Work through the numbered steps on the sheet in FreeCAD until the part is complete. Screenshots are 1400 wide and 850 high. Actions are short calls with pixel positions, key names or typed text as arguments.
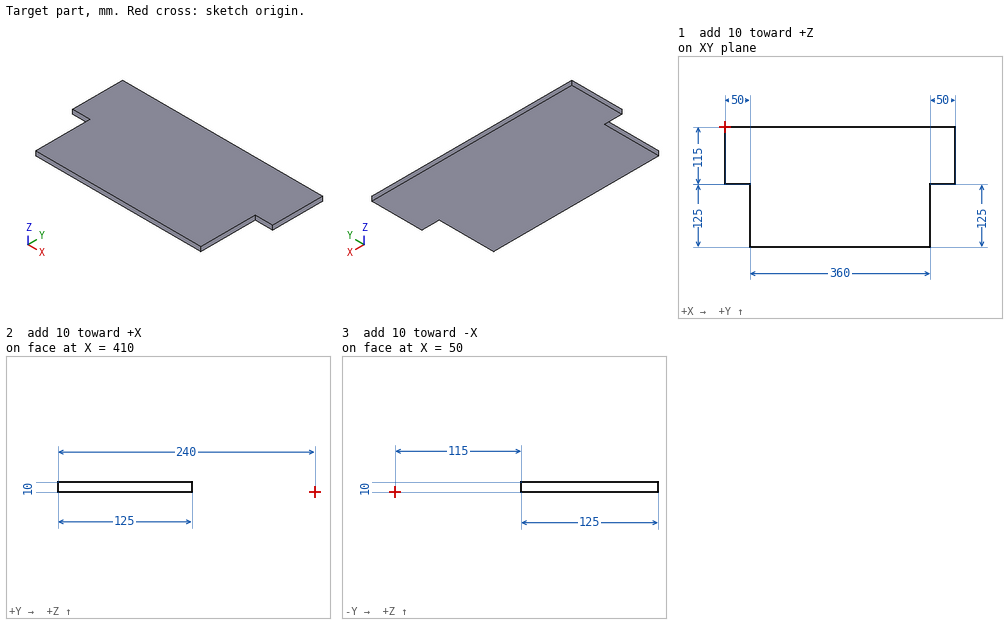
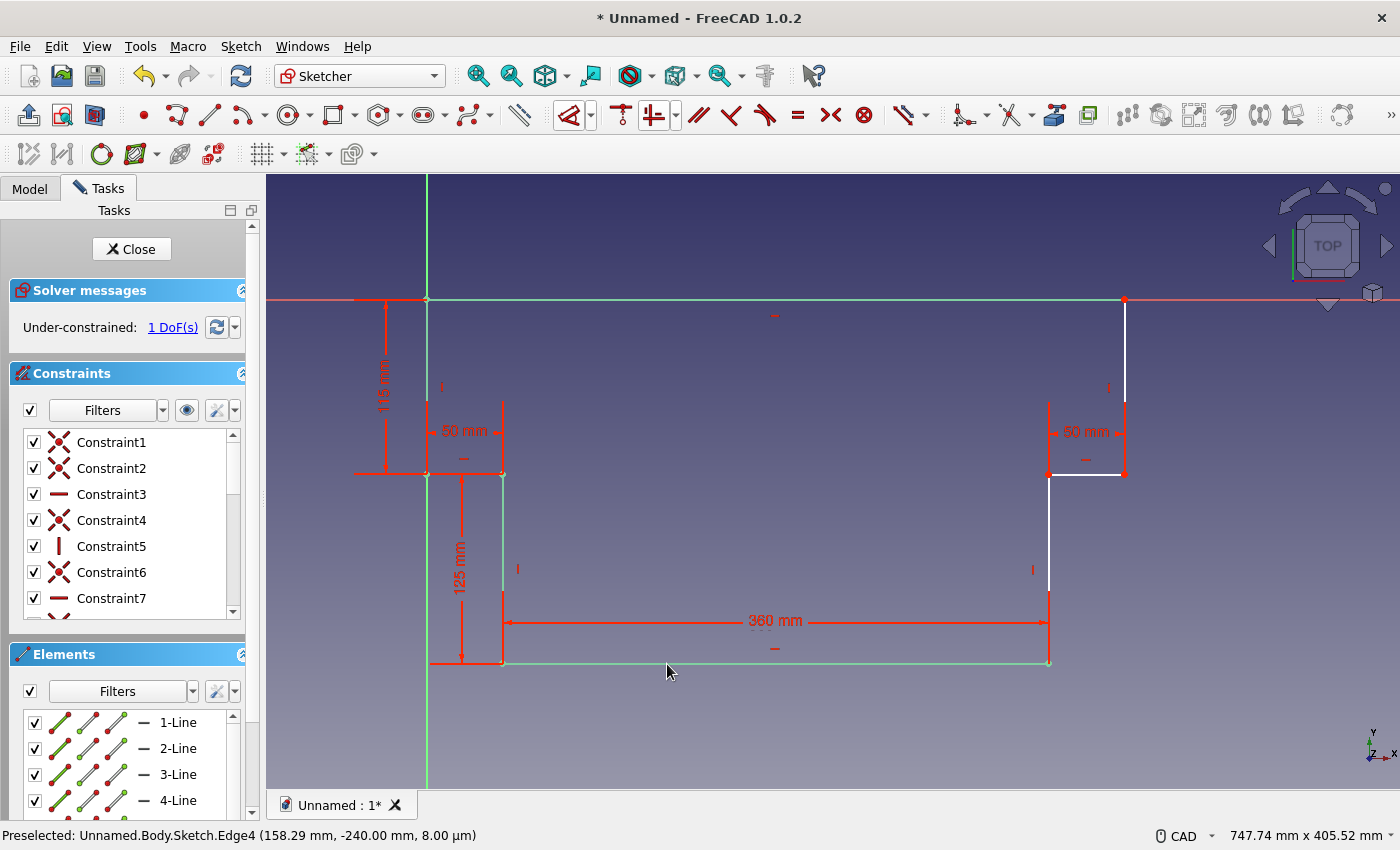
click(1049, 607)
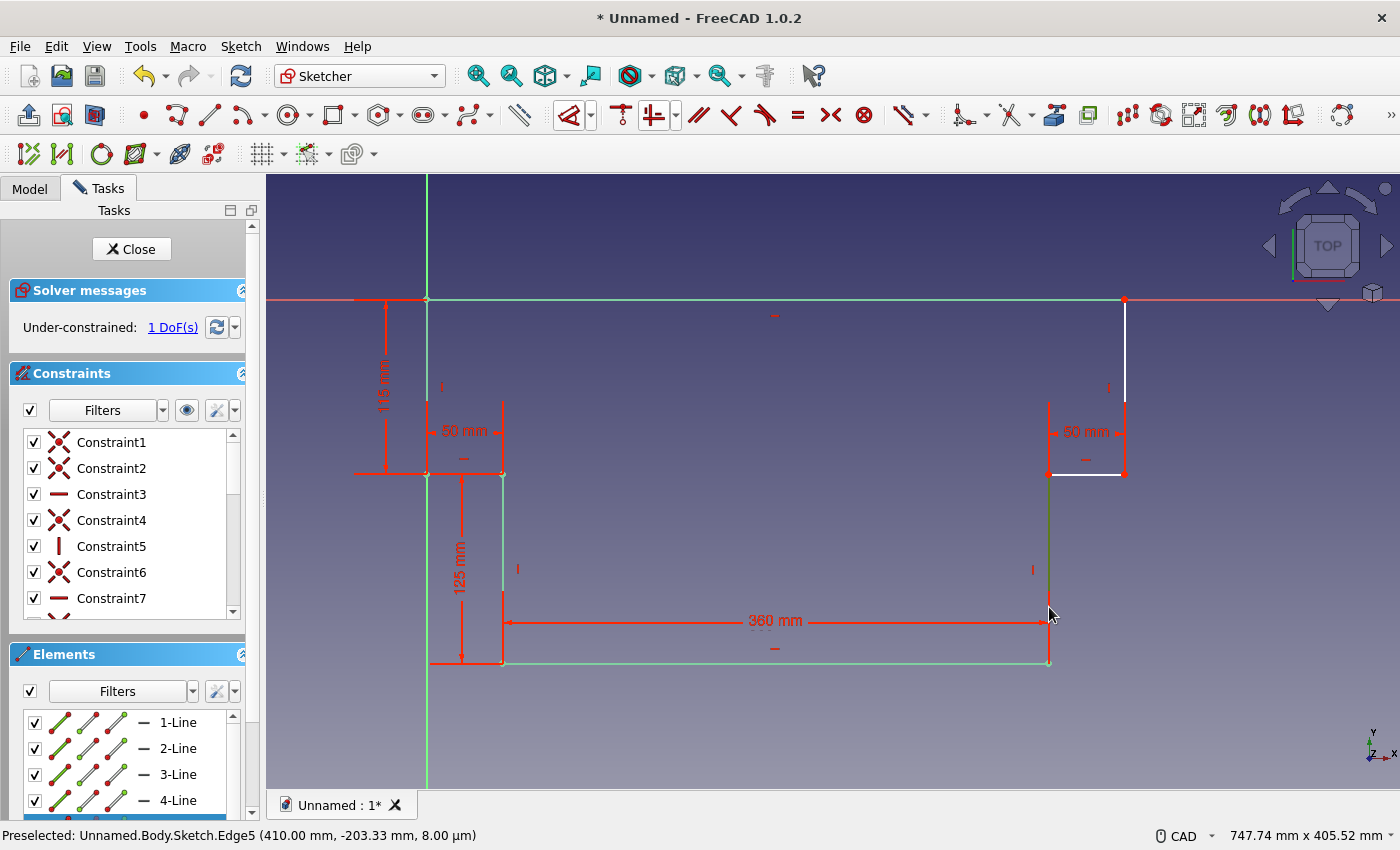
key(i)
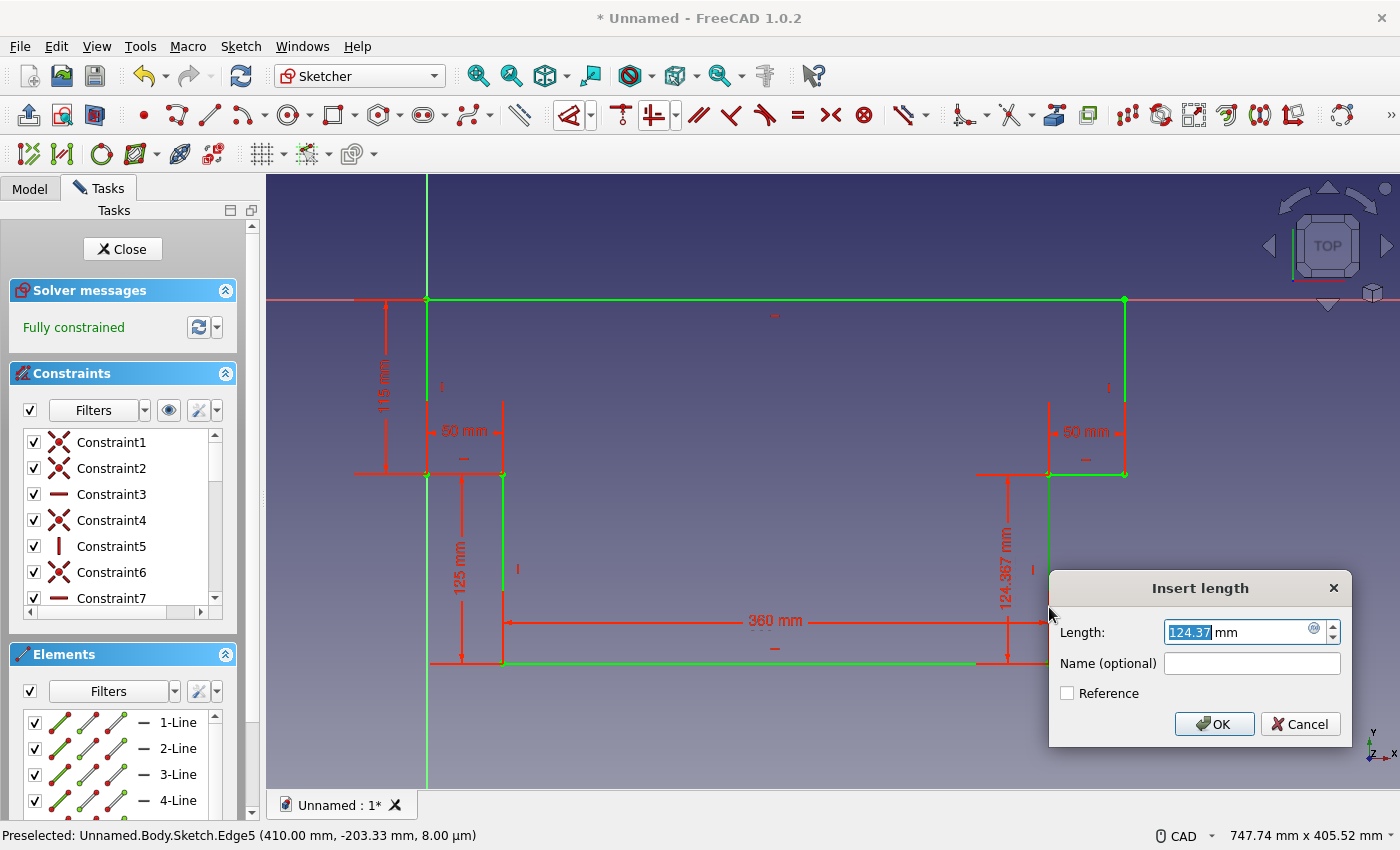
text(125)
key(Return)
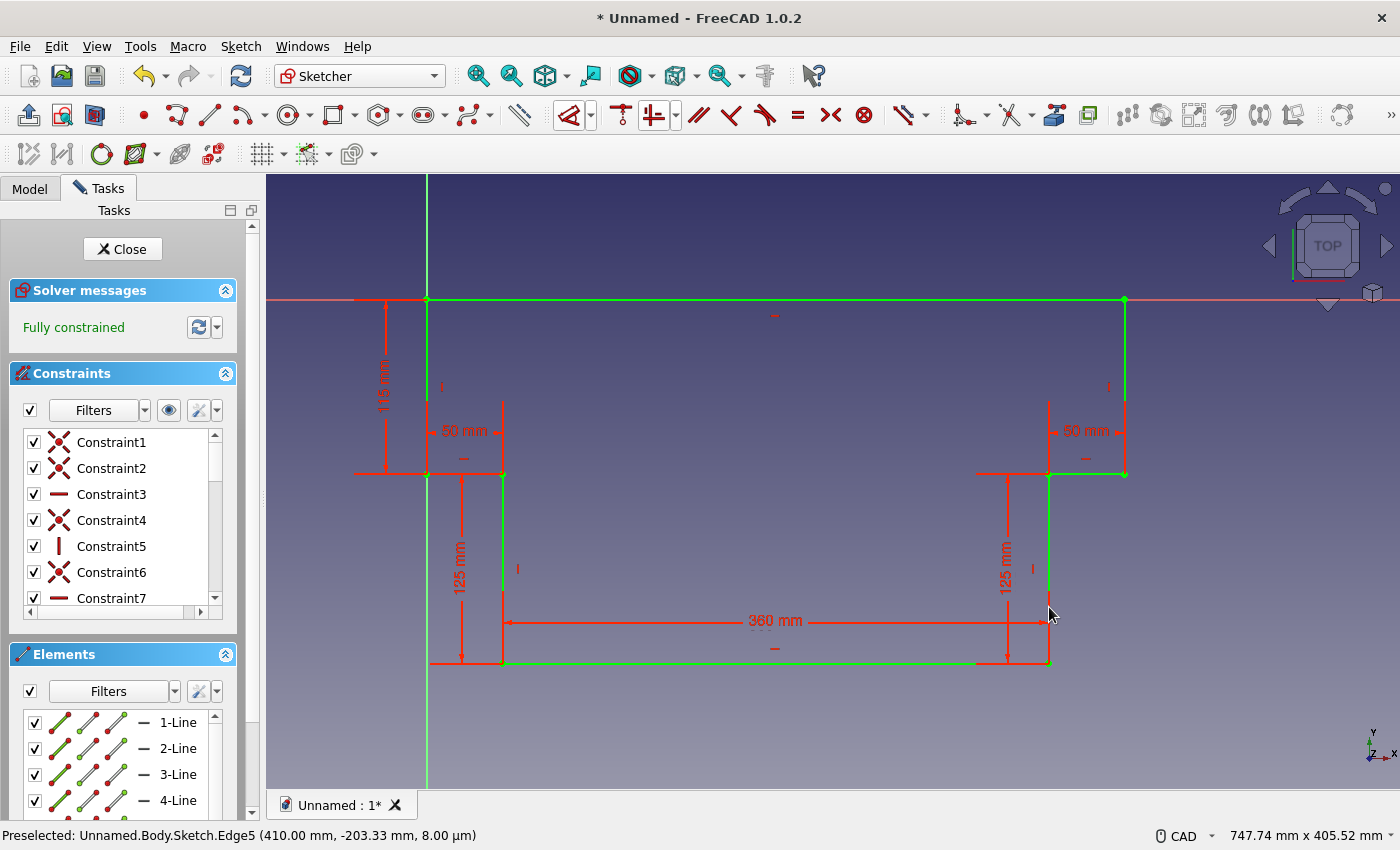
click(123, 249)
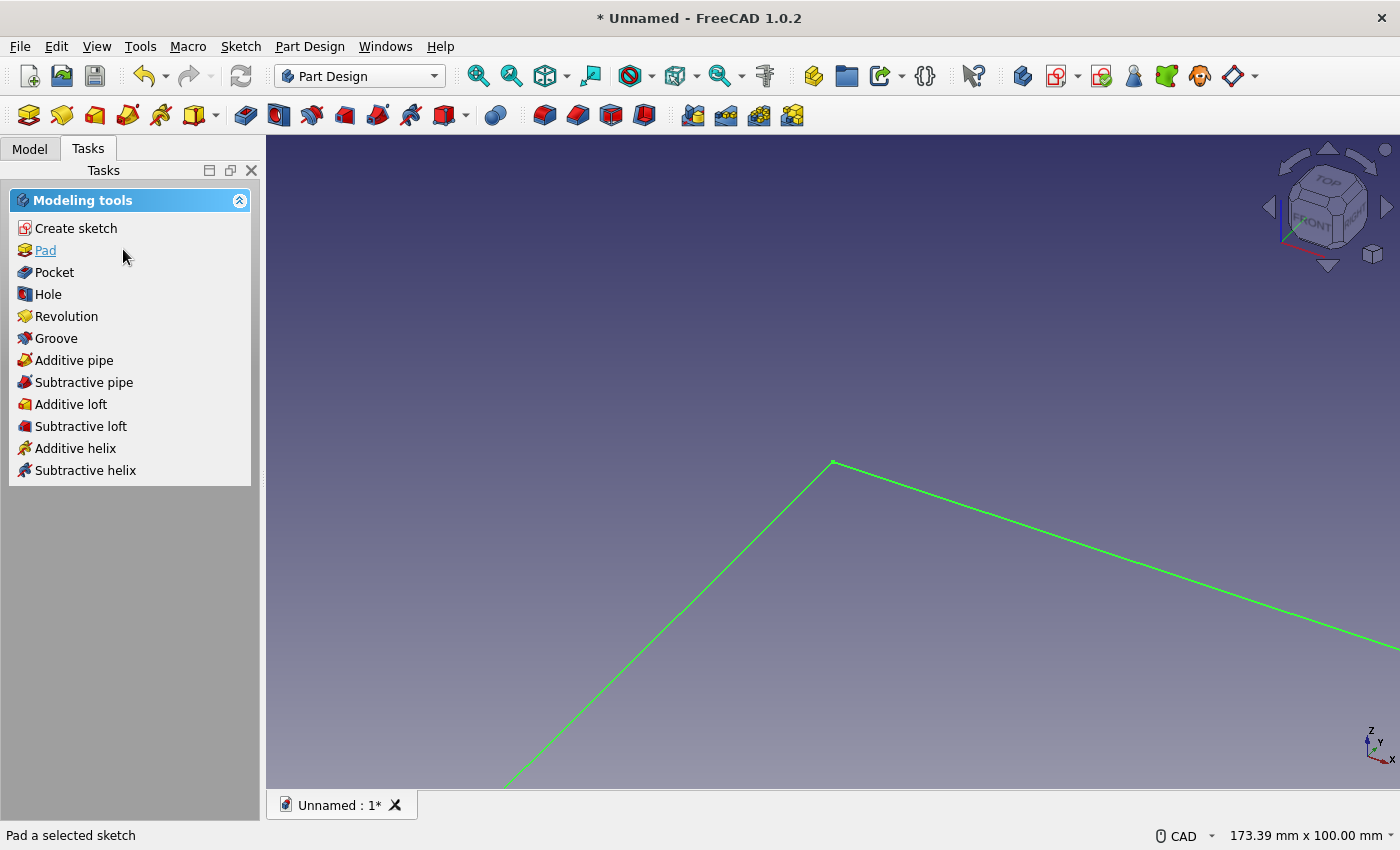
click(29, 116)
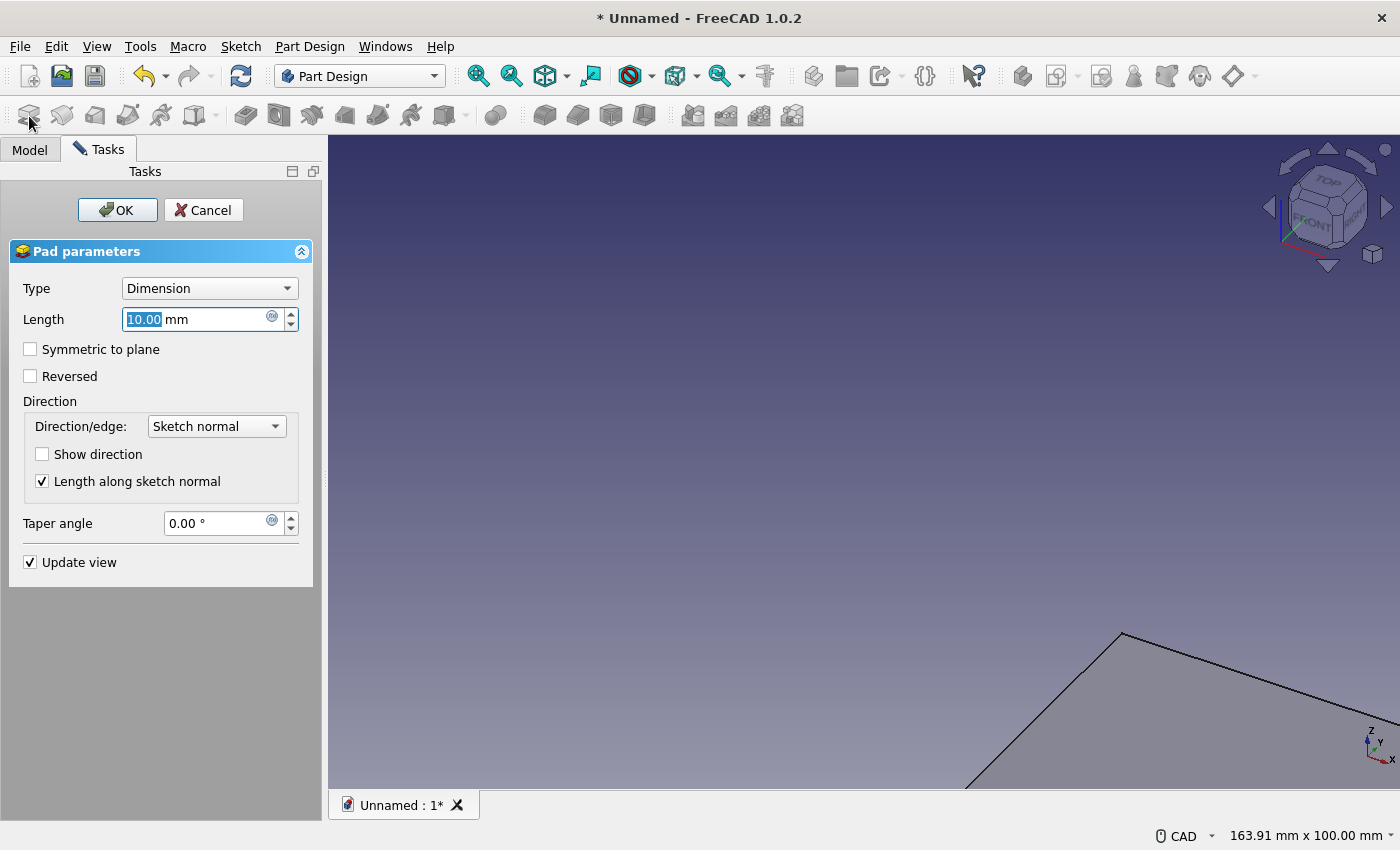
text(10)
key(Tab)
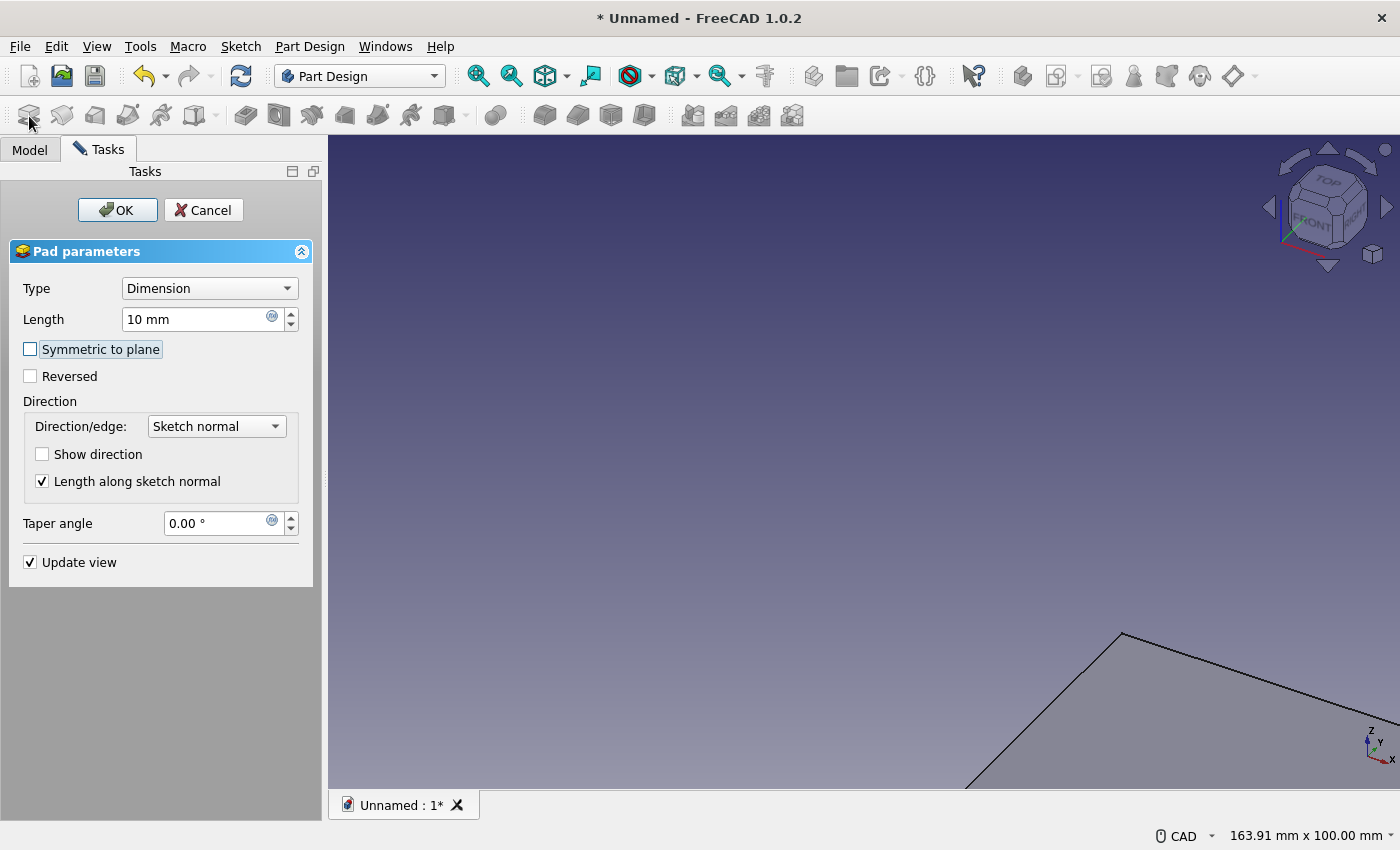
click(118, 210)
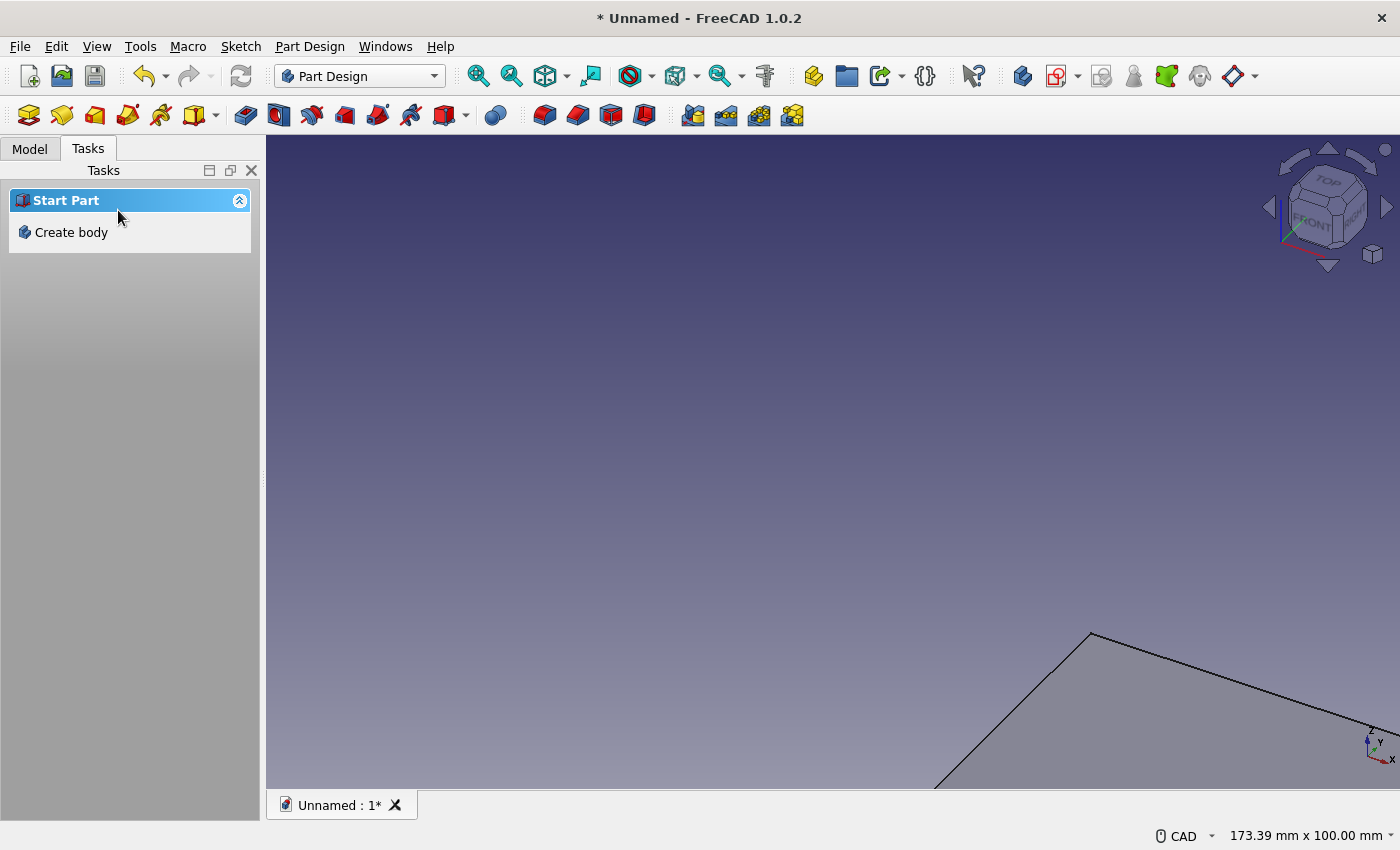
click(479, 76)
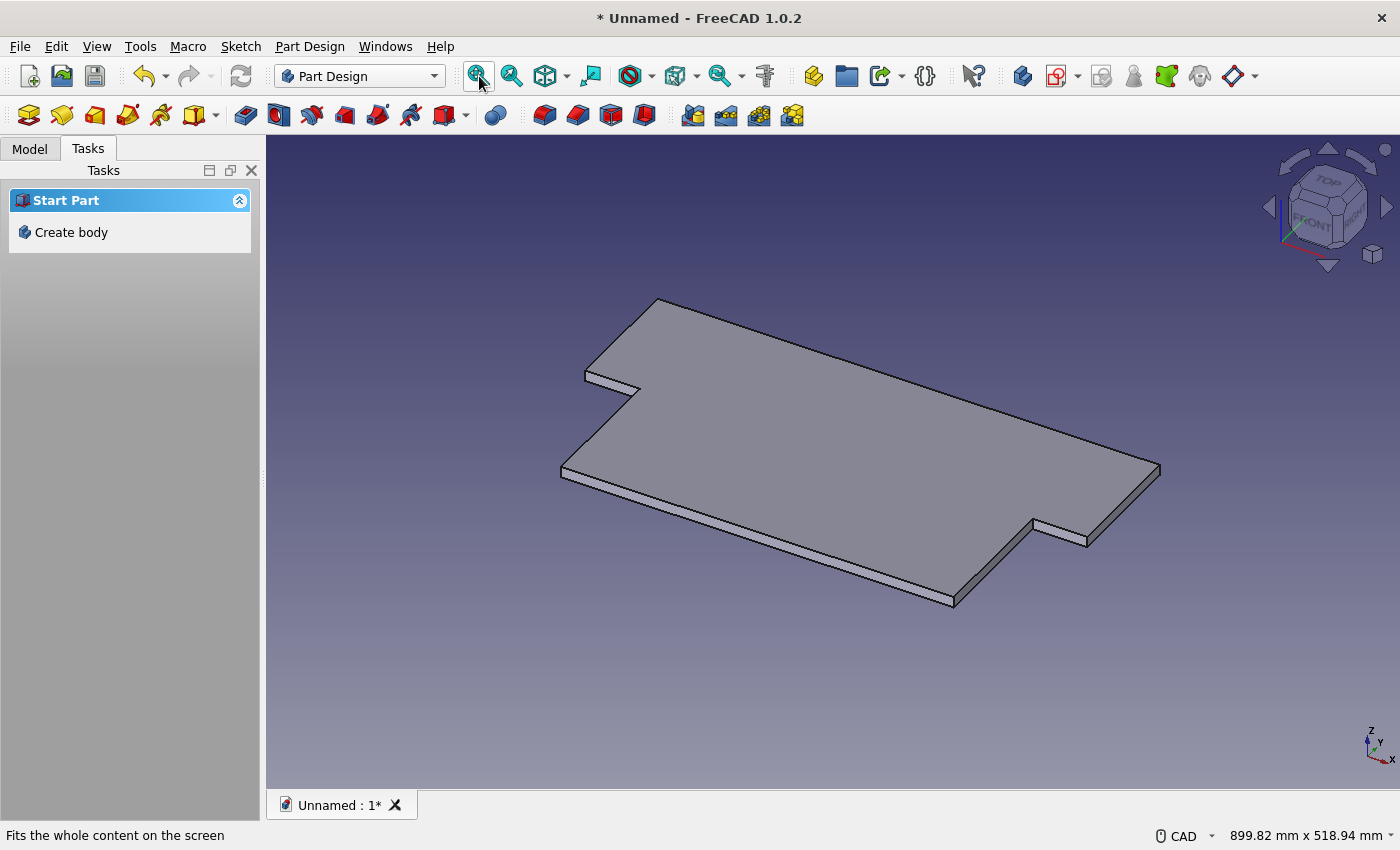
scroll(1027, 529, up, 4)